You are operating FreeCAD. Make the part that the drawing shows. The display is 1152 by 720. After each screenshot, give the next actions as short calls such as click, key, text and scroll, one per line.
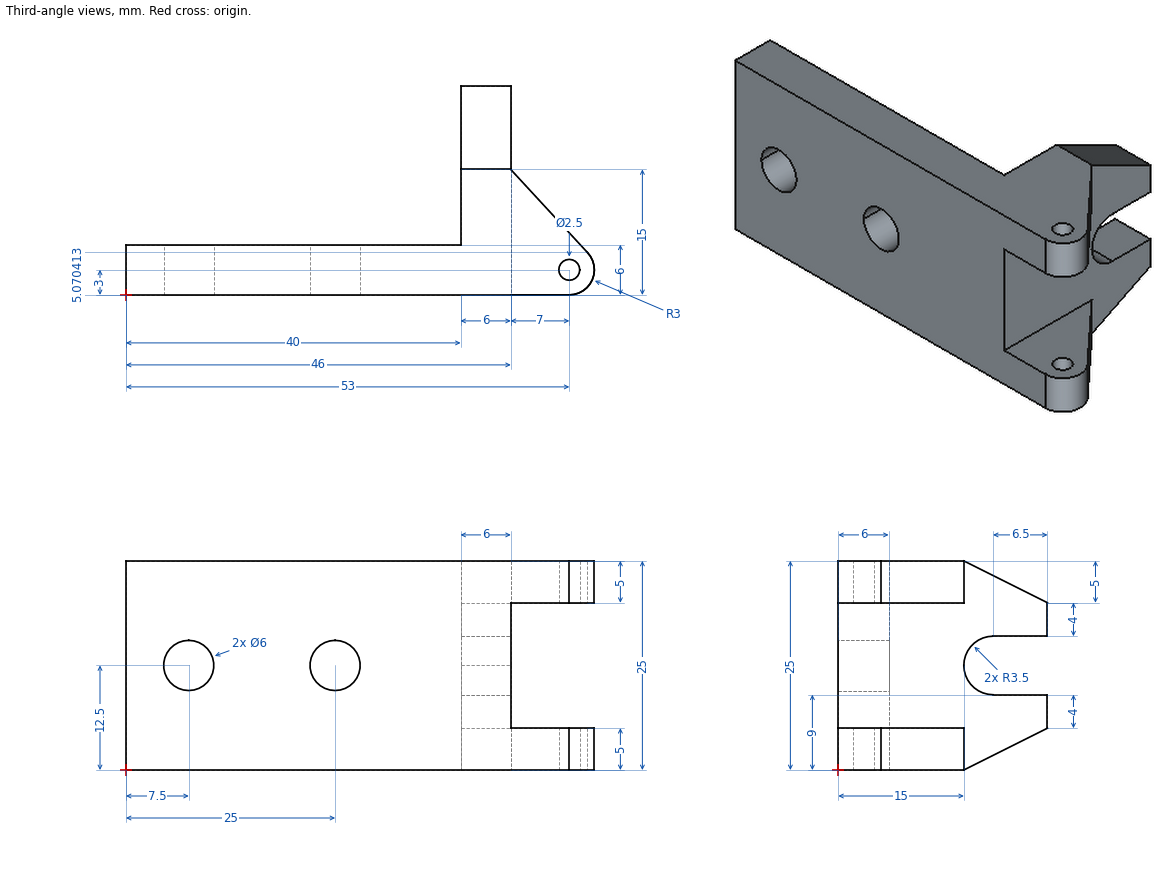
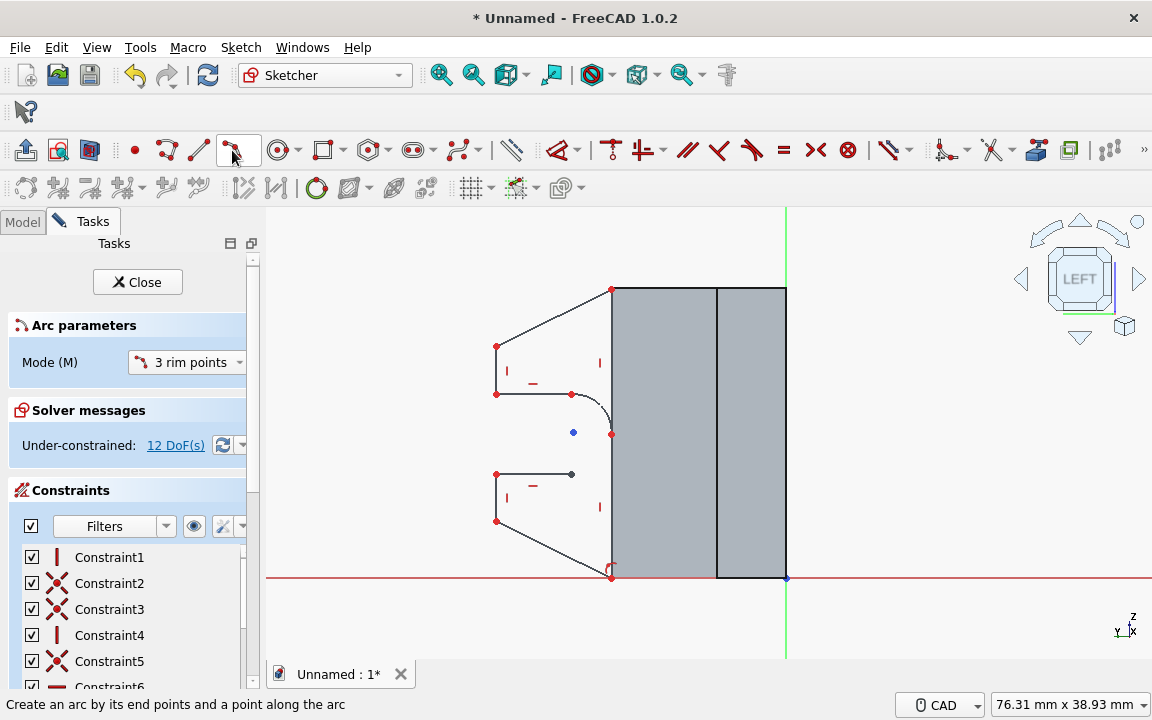
click(612, 434)
click(571, 474)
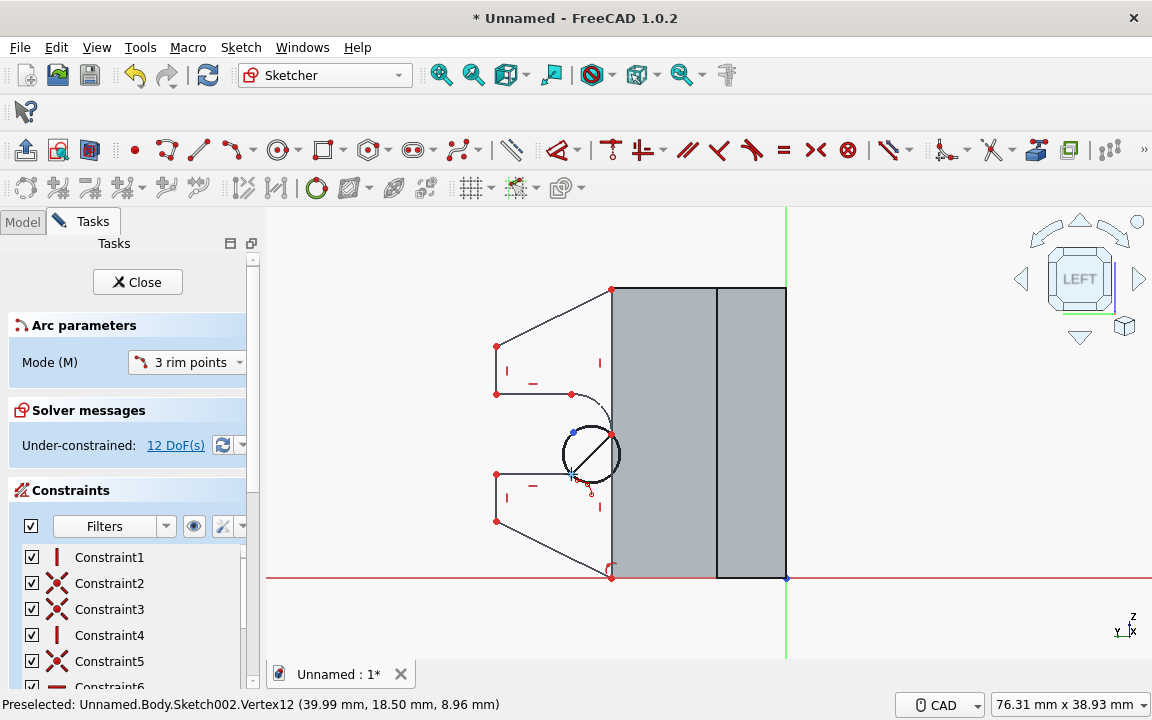
scroll(600, 462, up, 2)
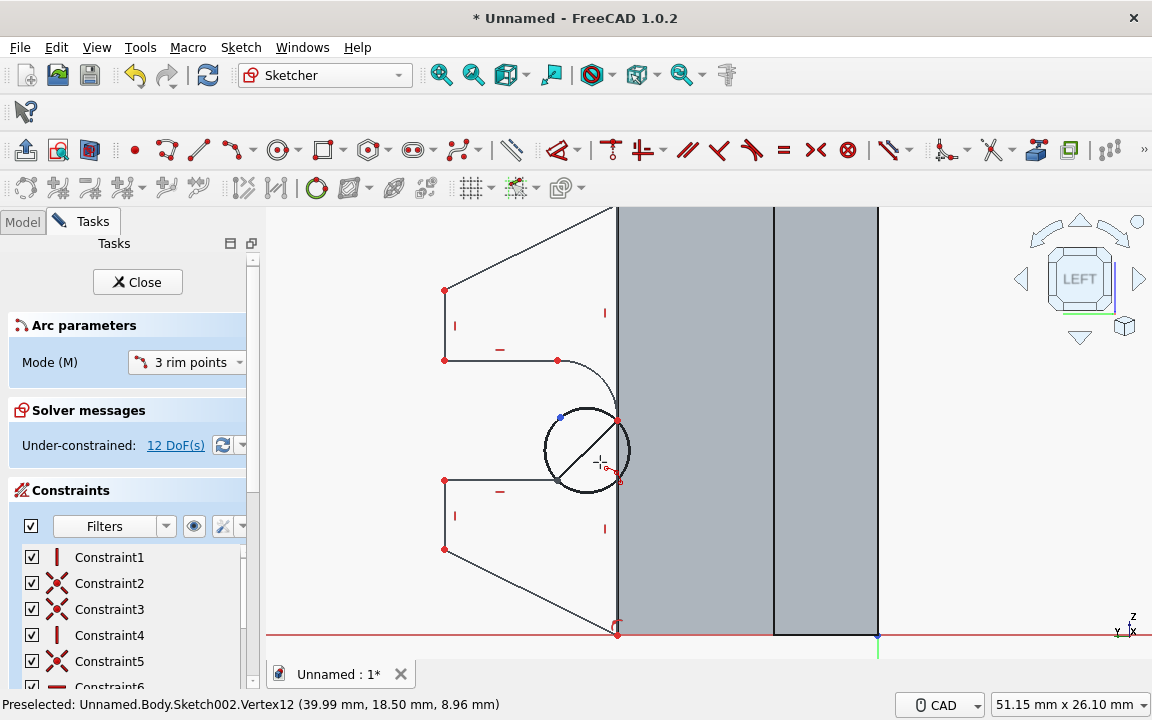
click(600, 462)
key(Escape)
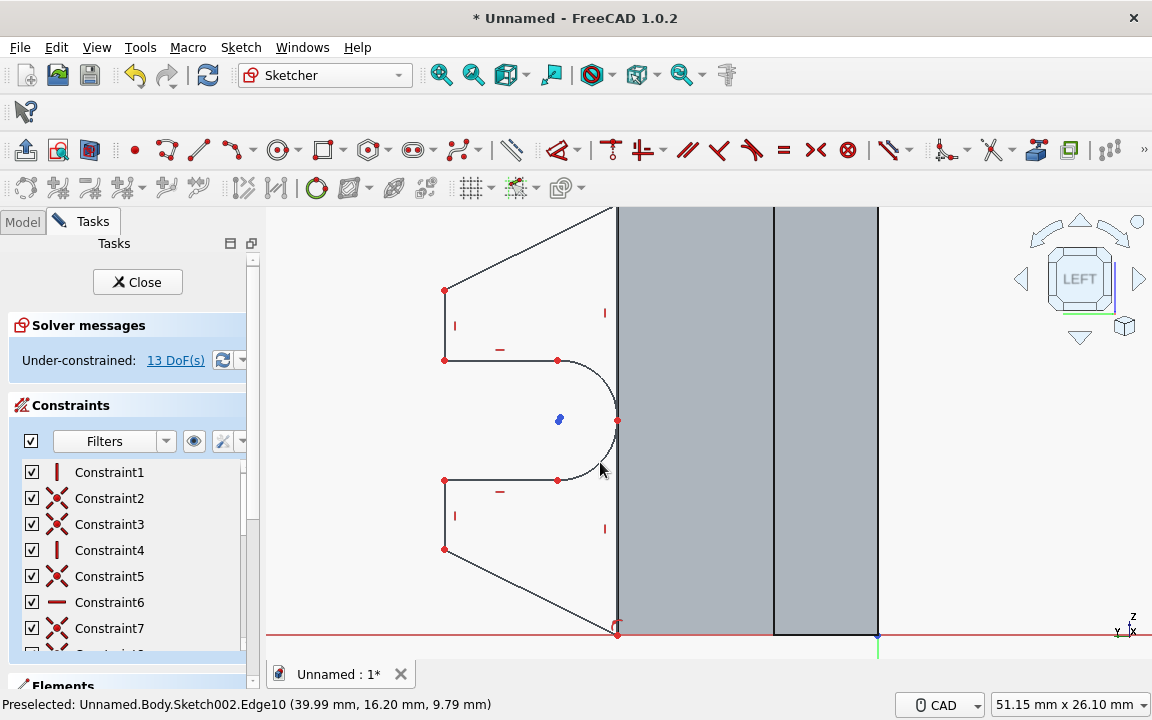
click(617, 356)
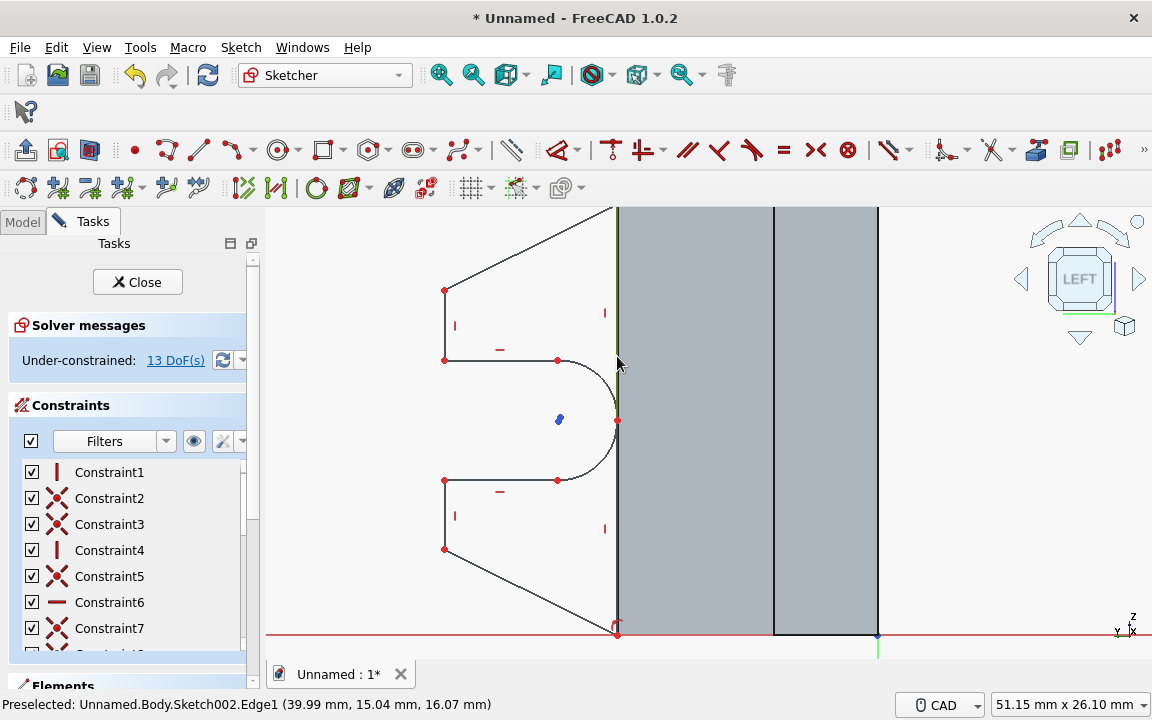
click(585, 366)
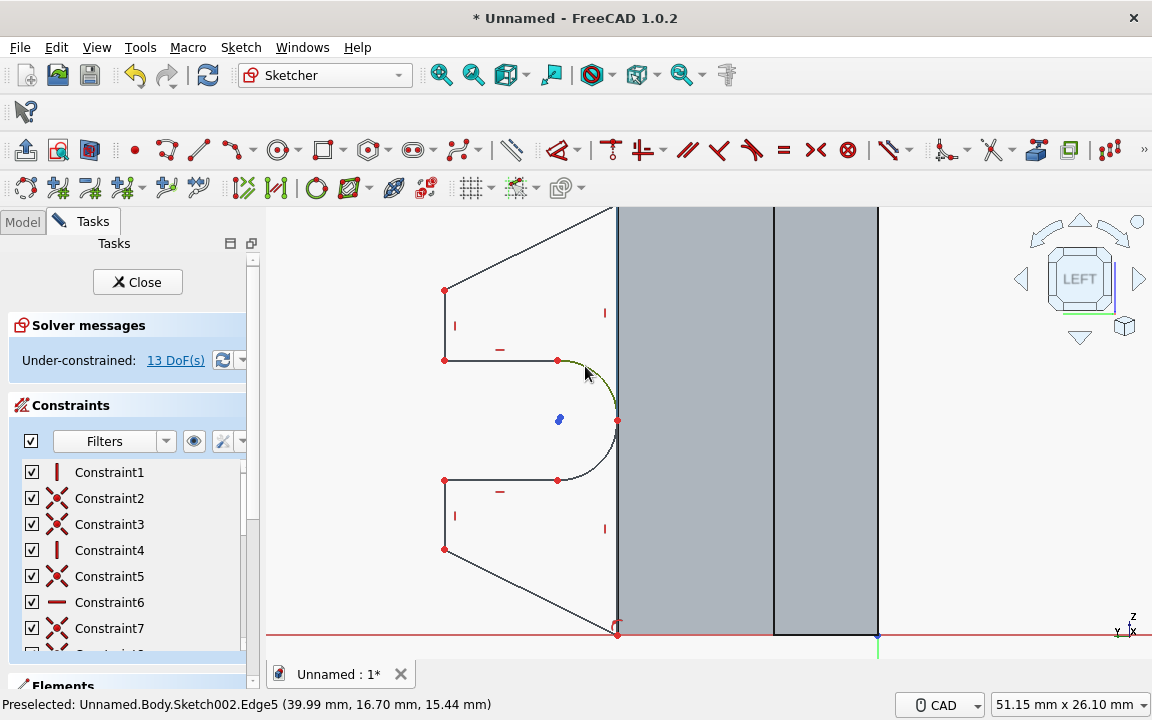
key(t)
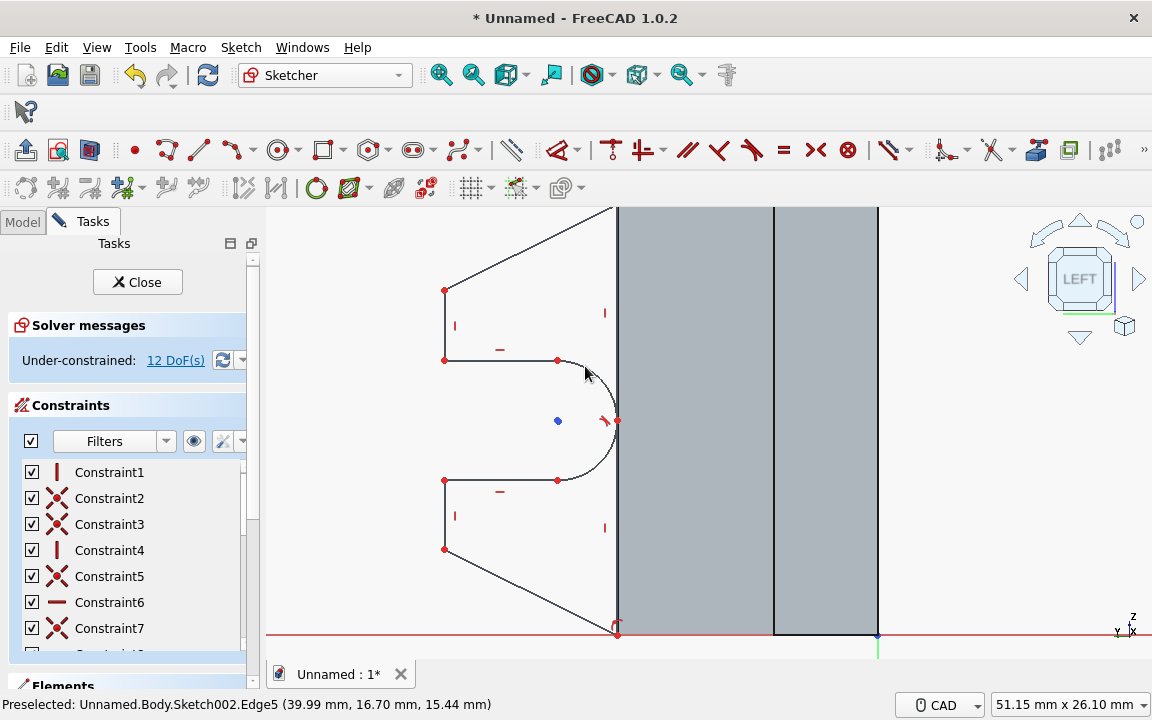
click(617, 356)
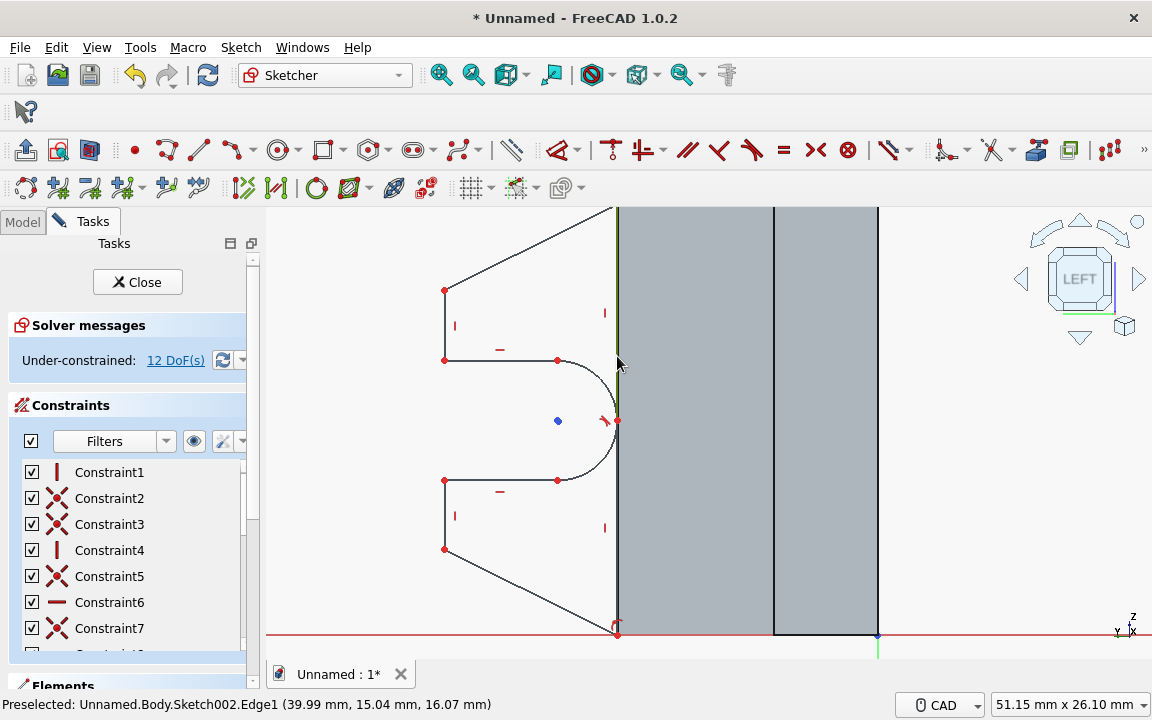
click(585, 474)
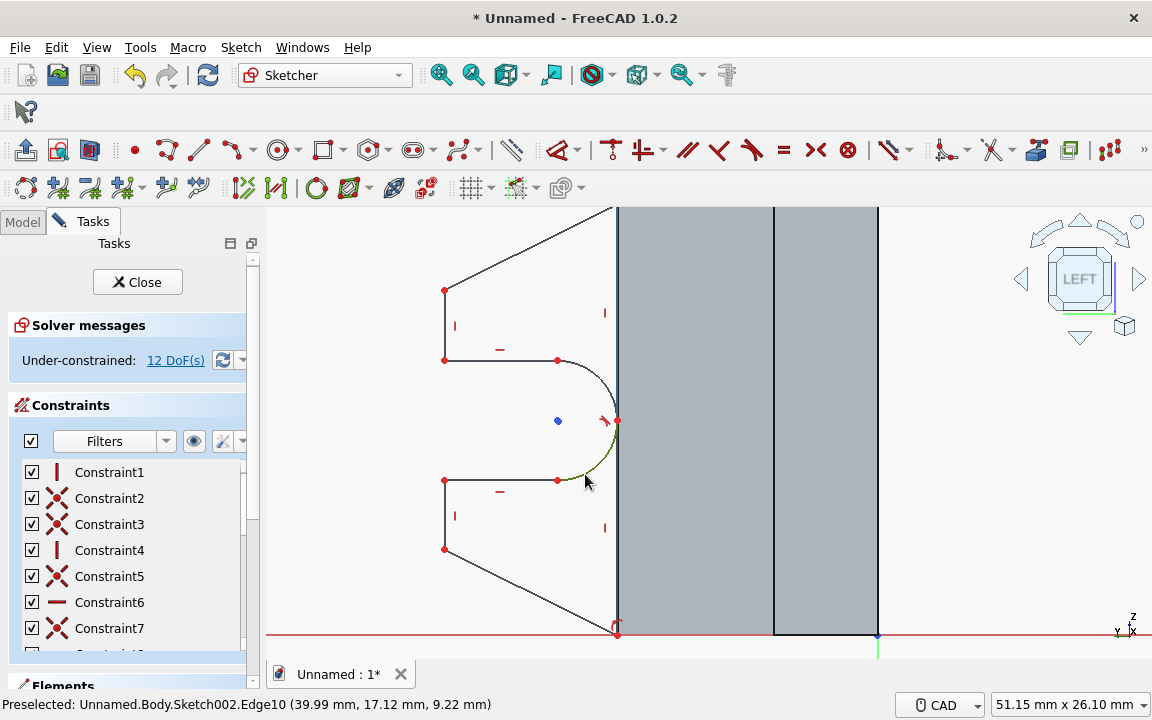
click(752, 150)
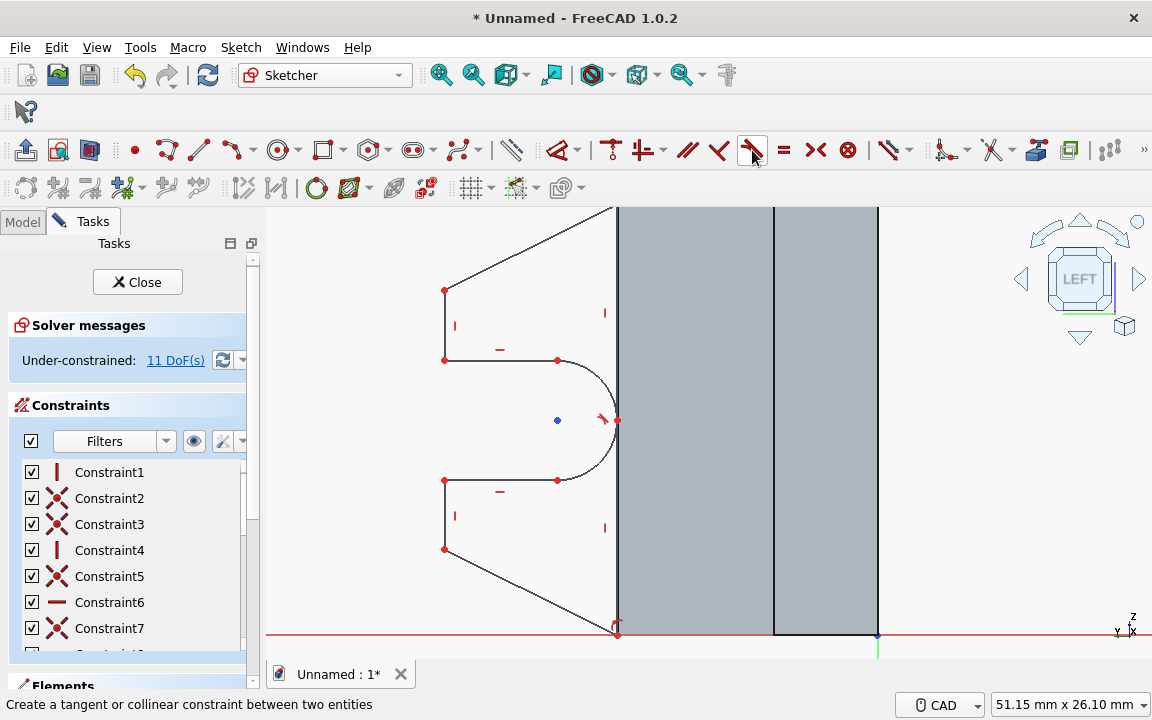
click(478, 361)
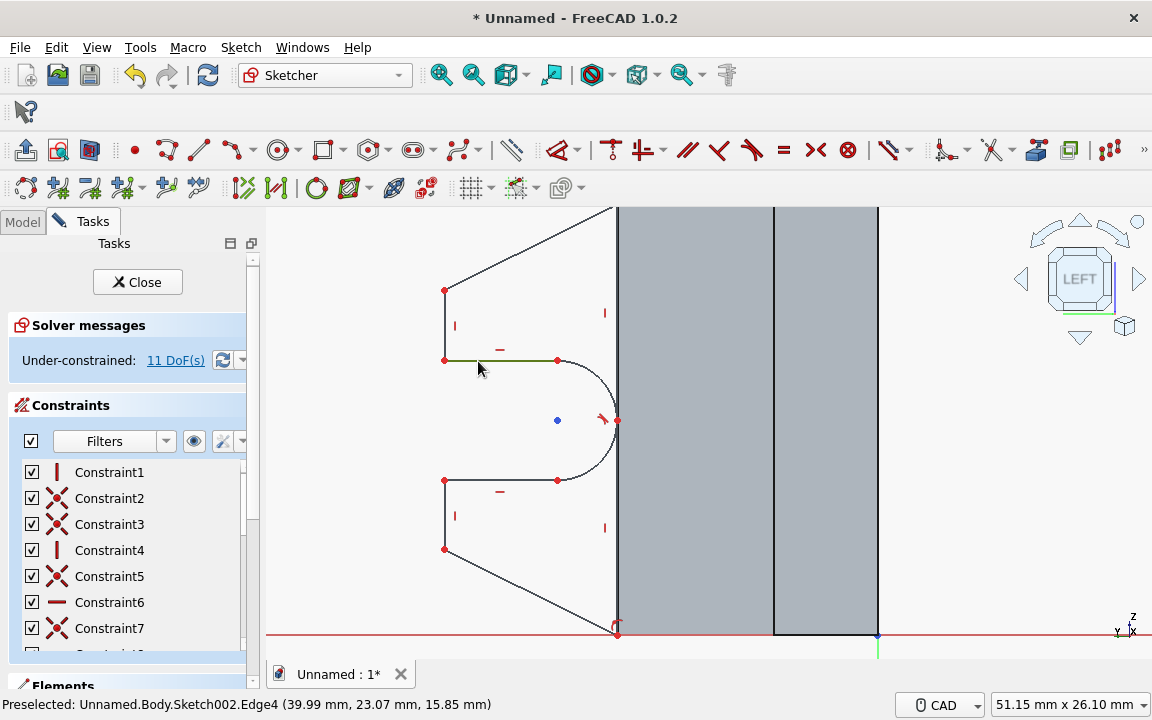
click(584, 367)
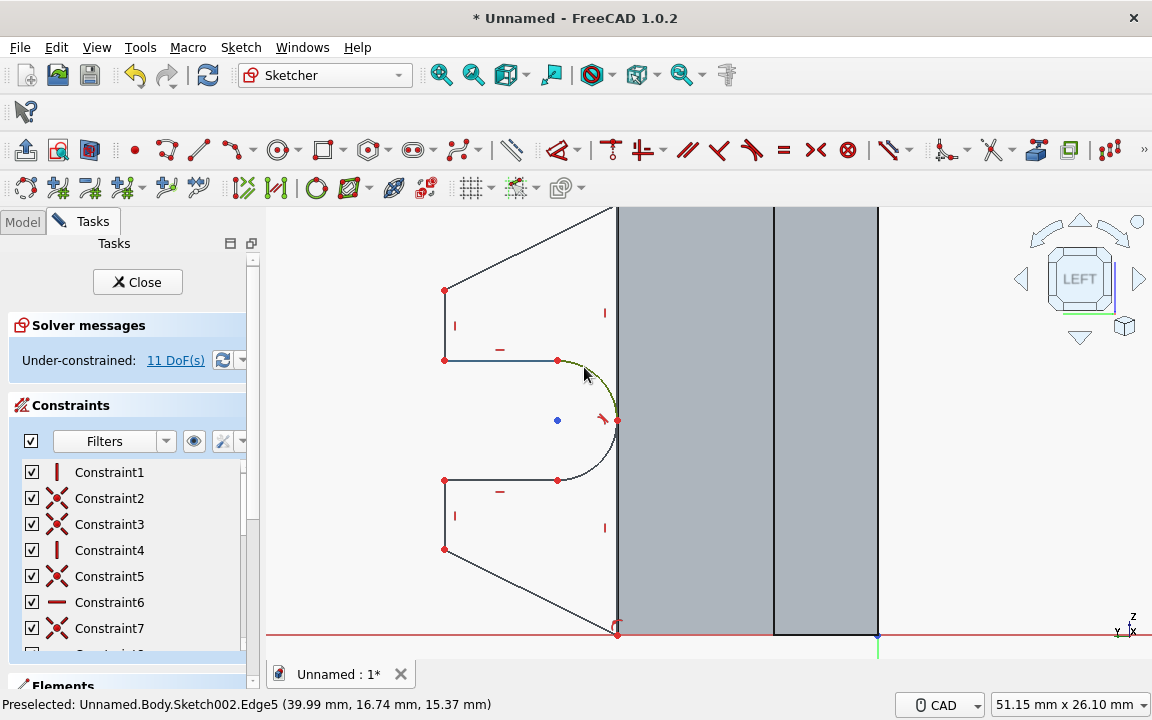
key(t)